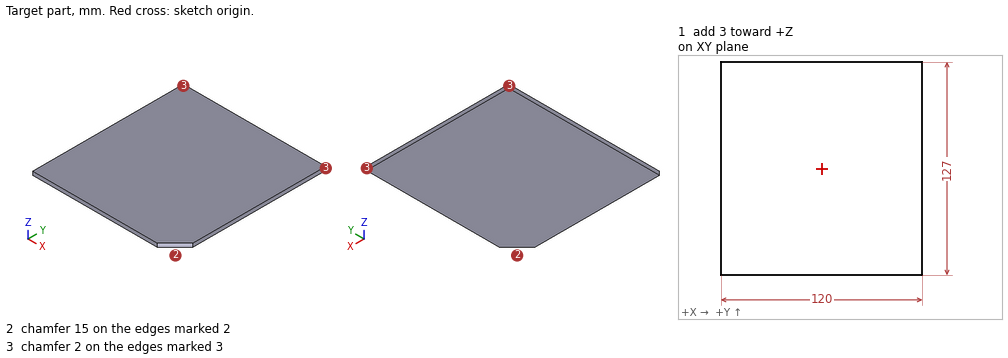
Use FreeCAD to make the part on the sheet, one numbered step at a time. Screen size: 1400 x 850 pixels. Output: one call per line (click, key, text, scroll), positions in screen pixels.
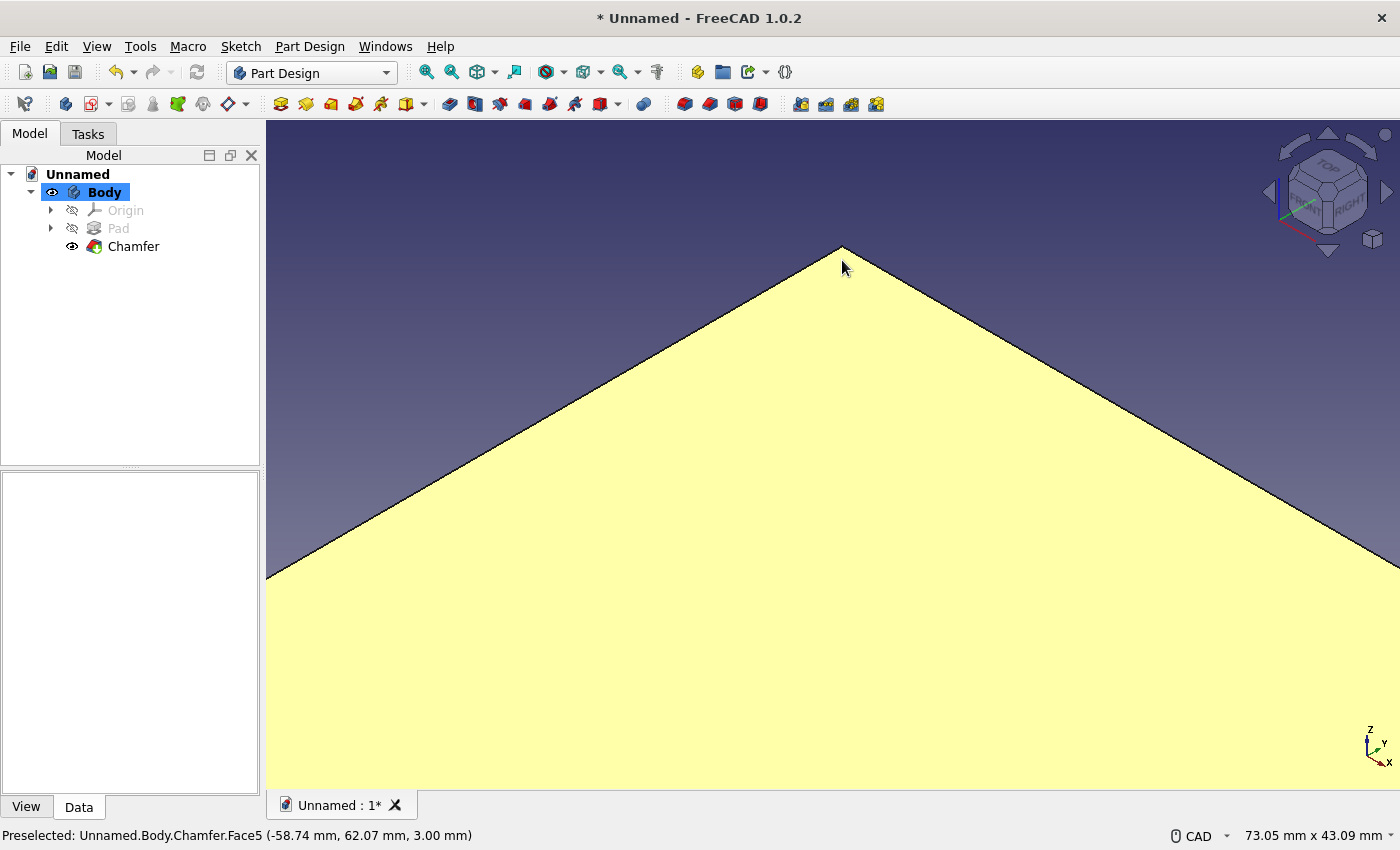
click(427, 72)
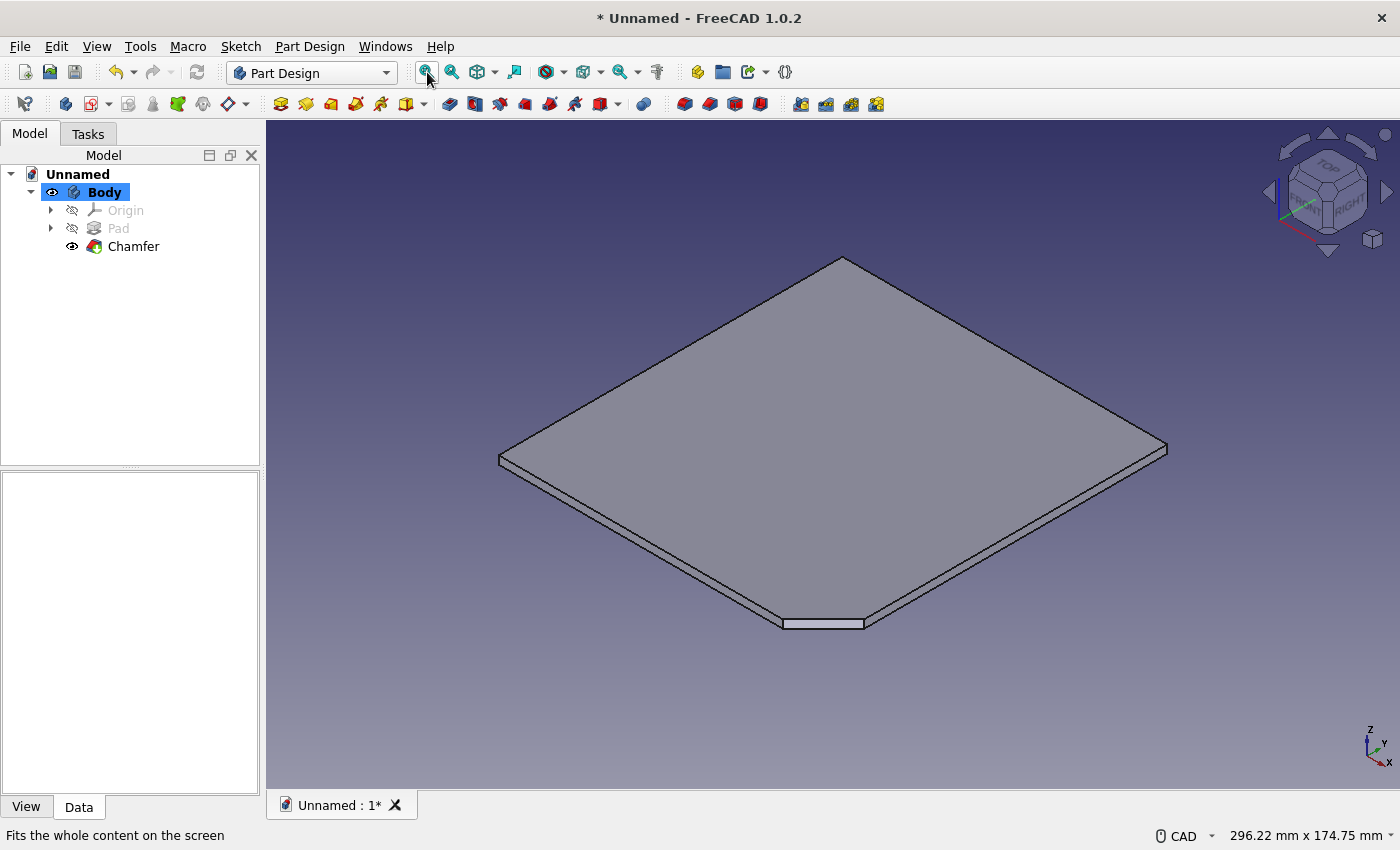
key(2)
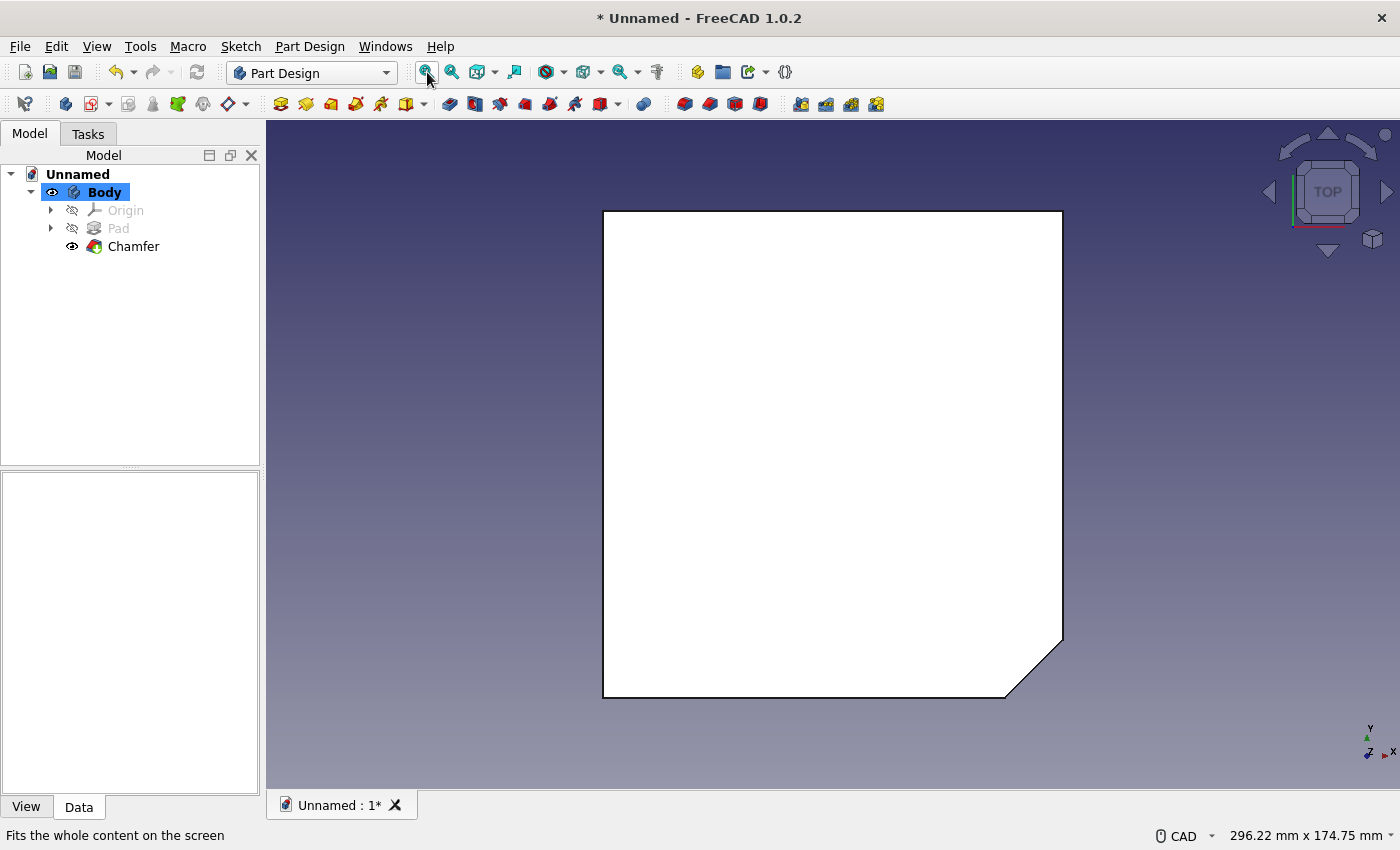
scroll(603, 210, up, 7)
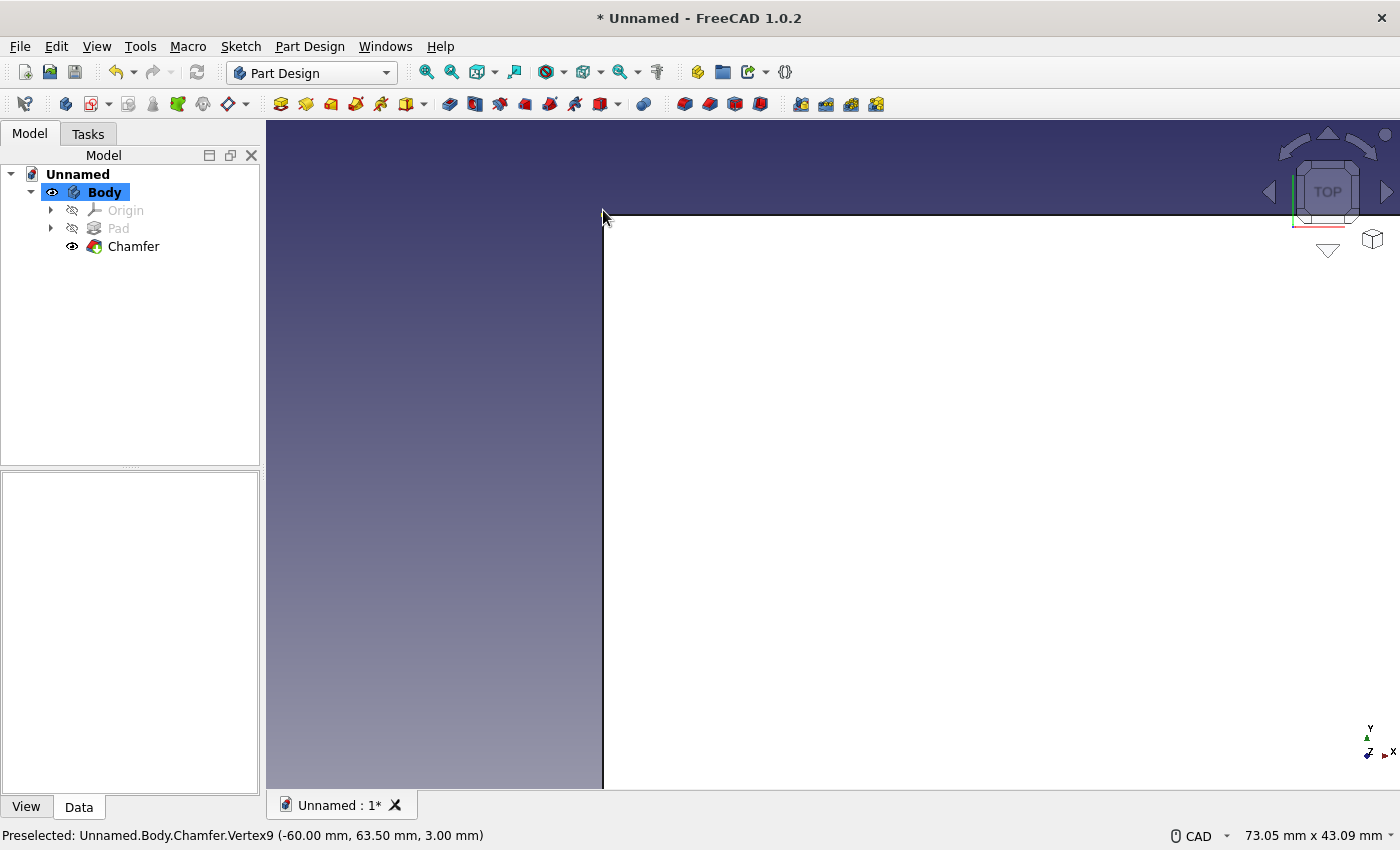
key(v)
key(f)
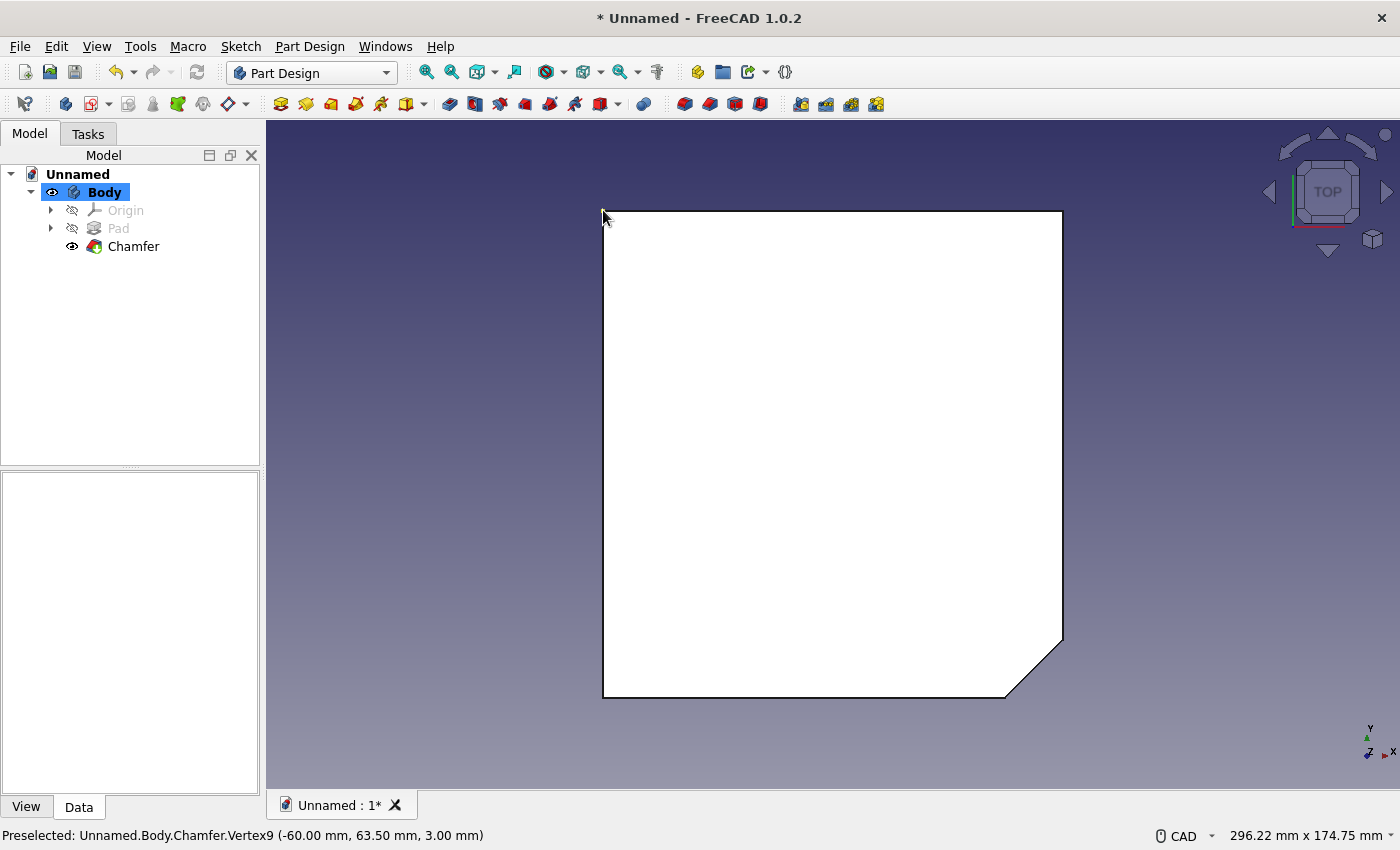
key(1)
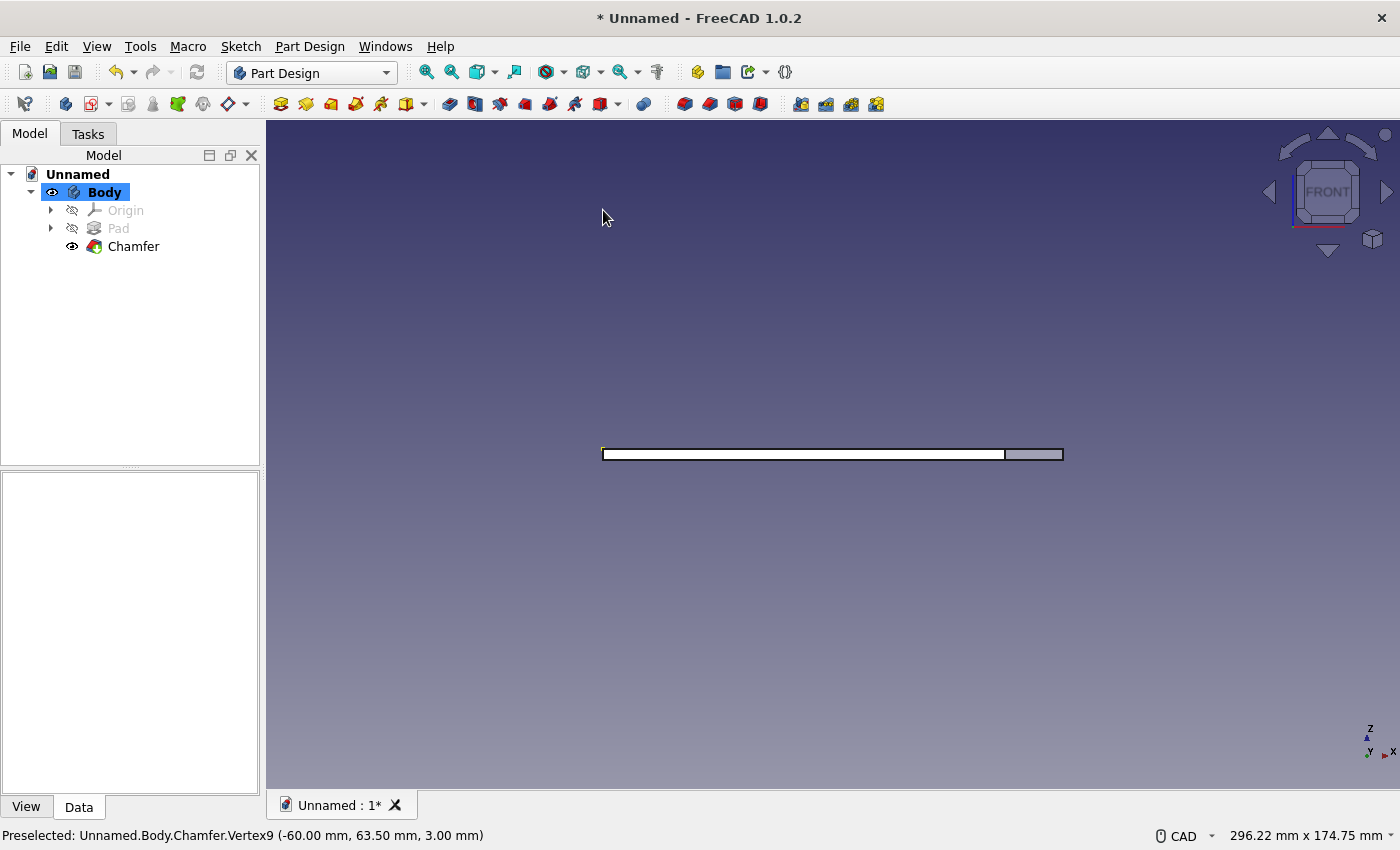
key(v)
key(f)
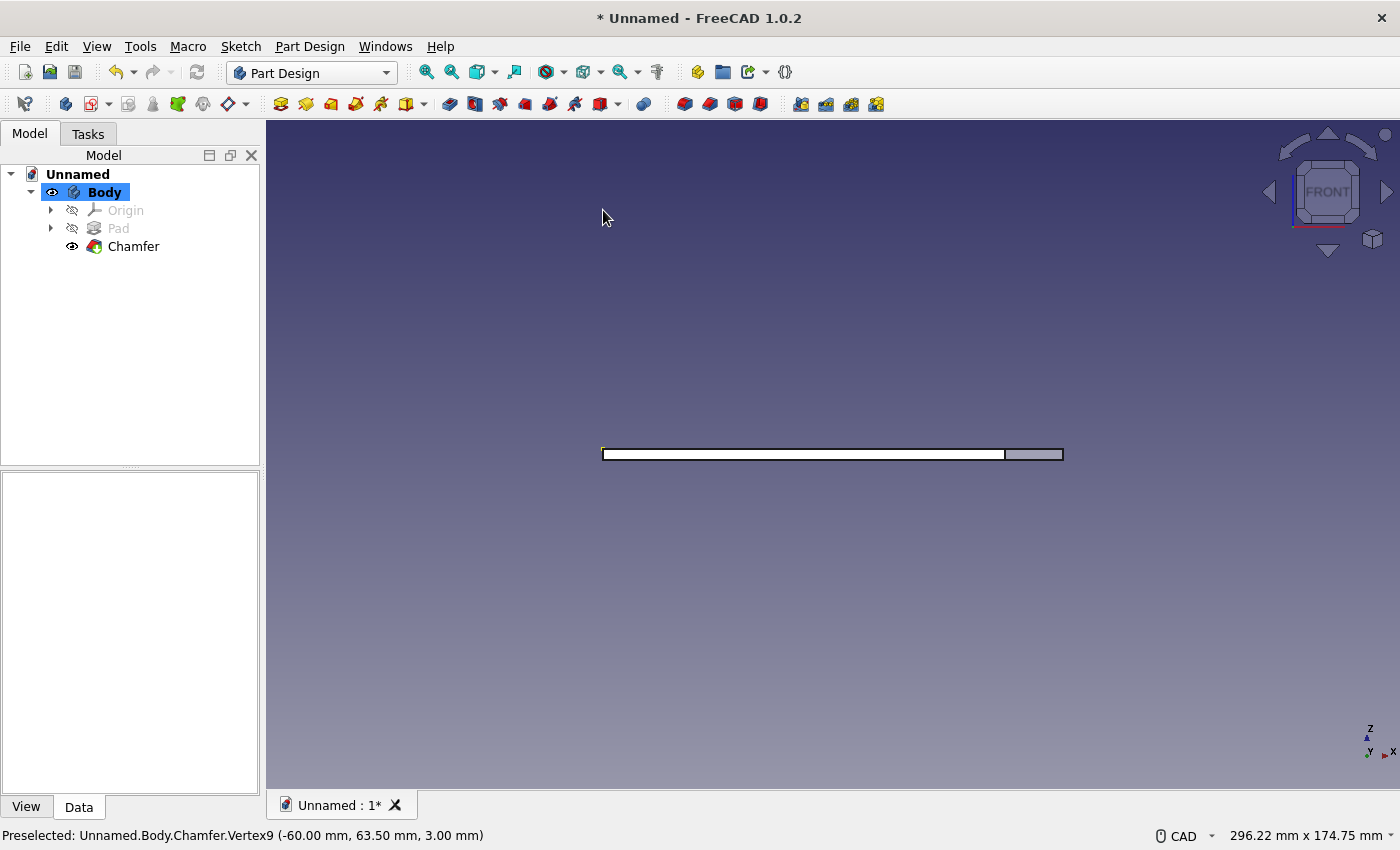
scroll(603, 454, up, 7)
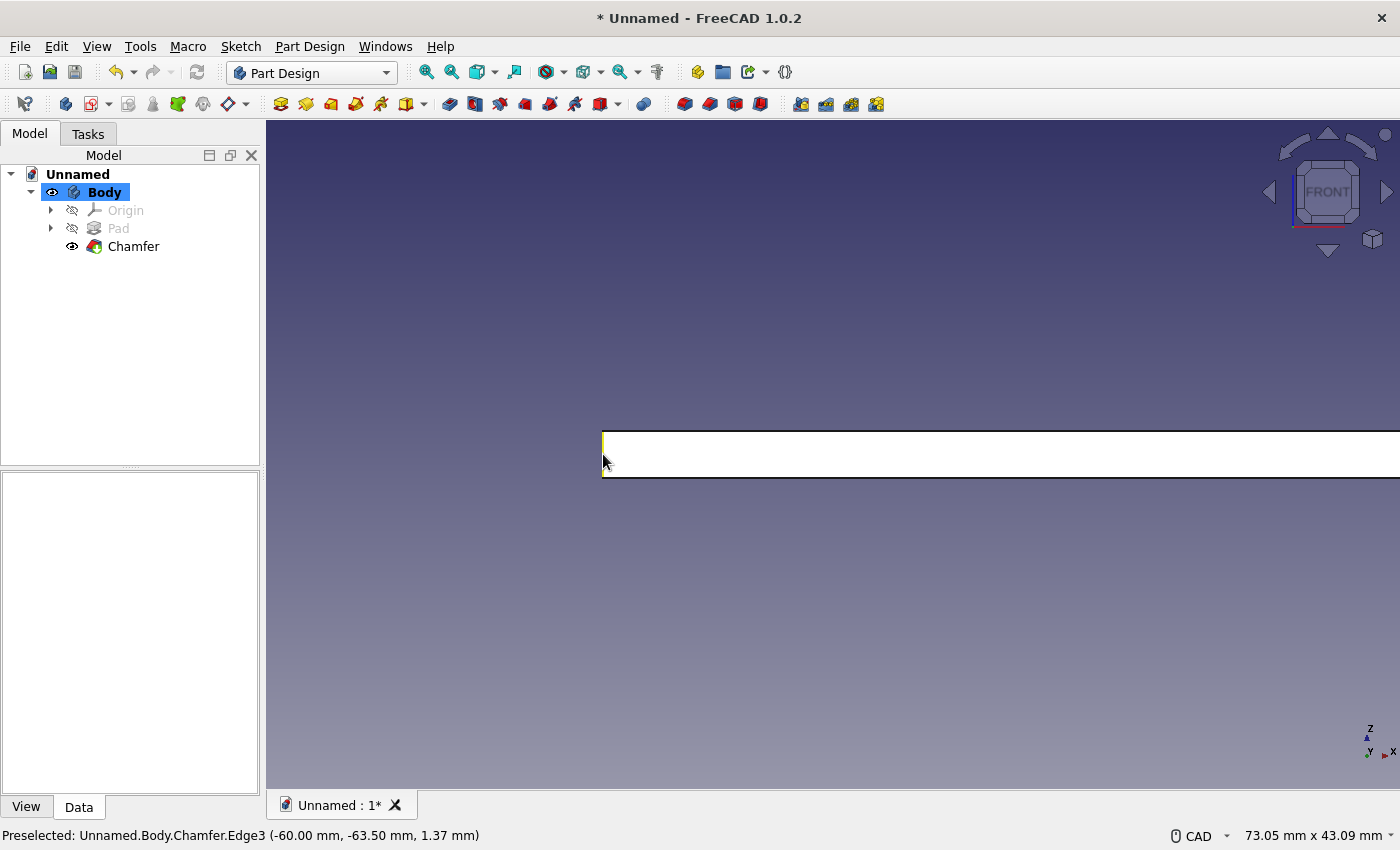
key(v)
key(f)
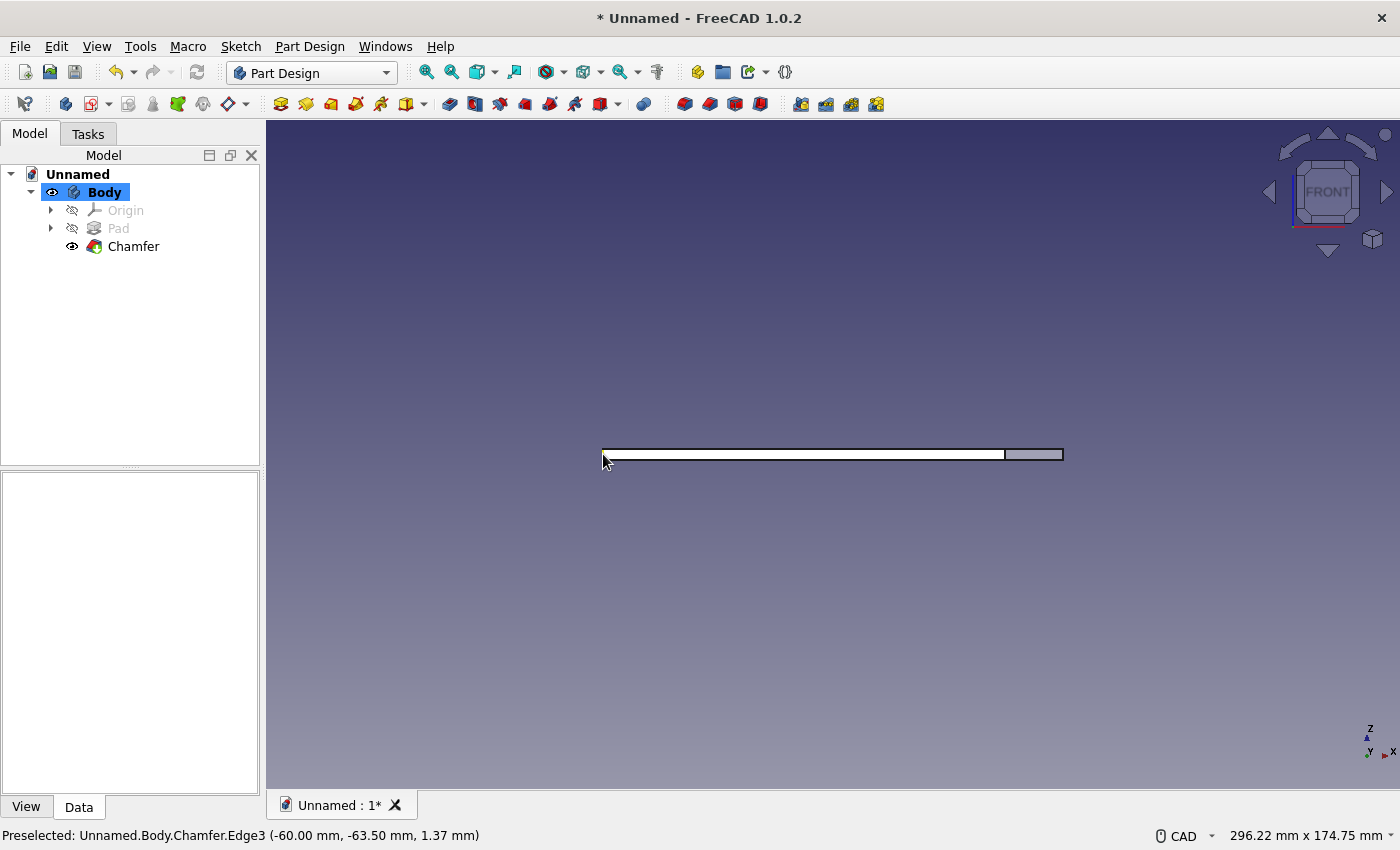
key(3)